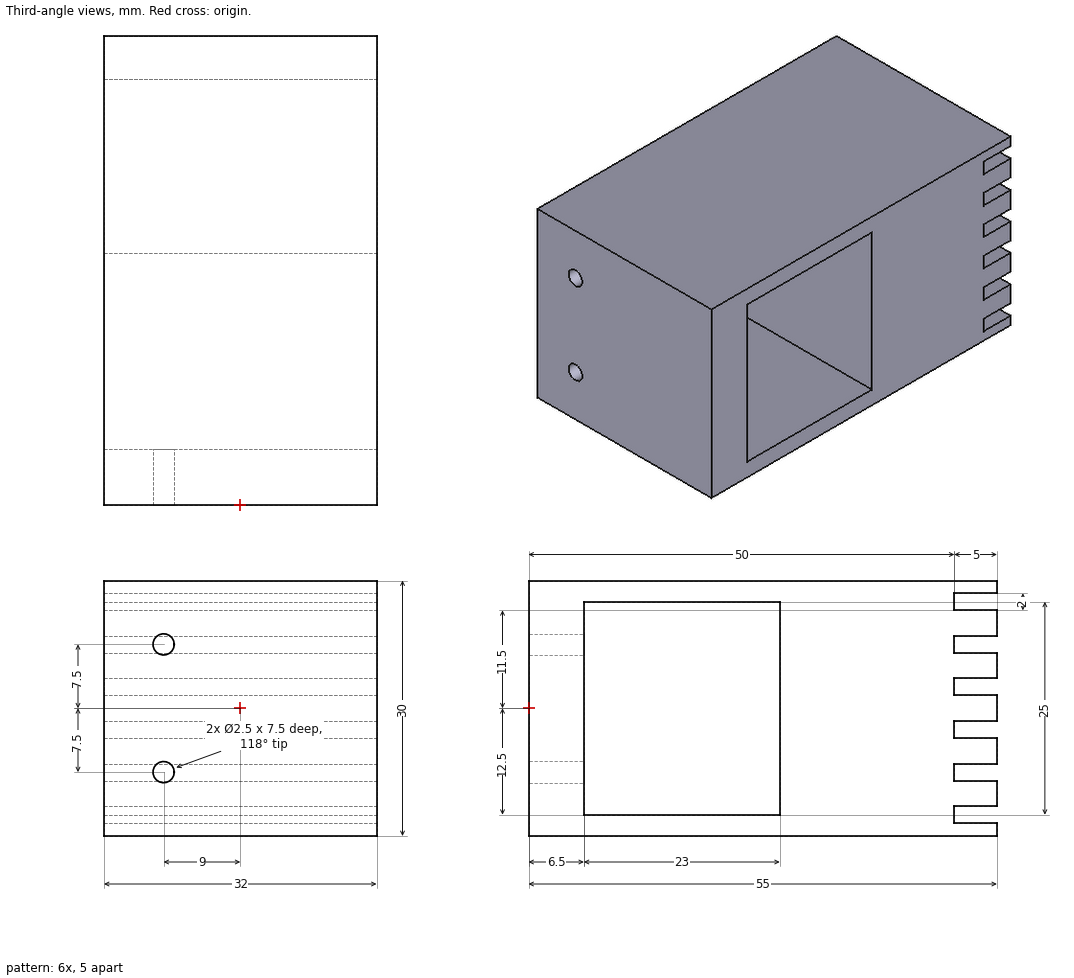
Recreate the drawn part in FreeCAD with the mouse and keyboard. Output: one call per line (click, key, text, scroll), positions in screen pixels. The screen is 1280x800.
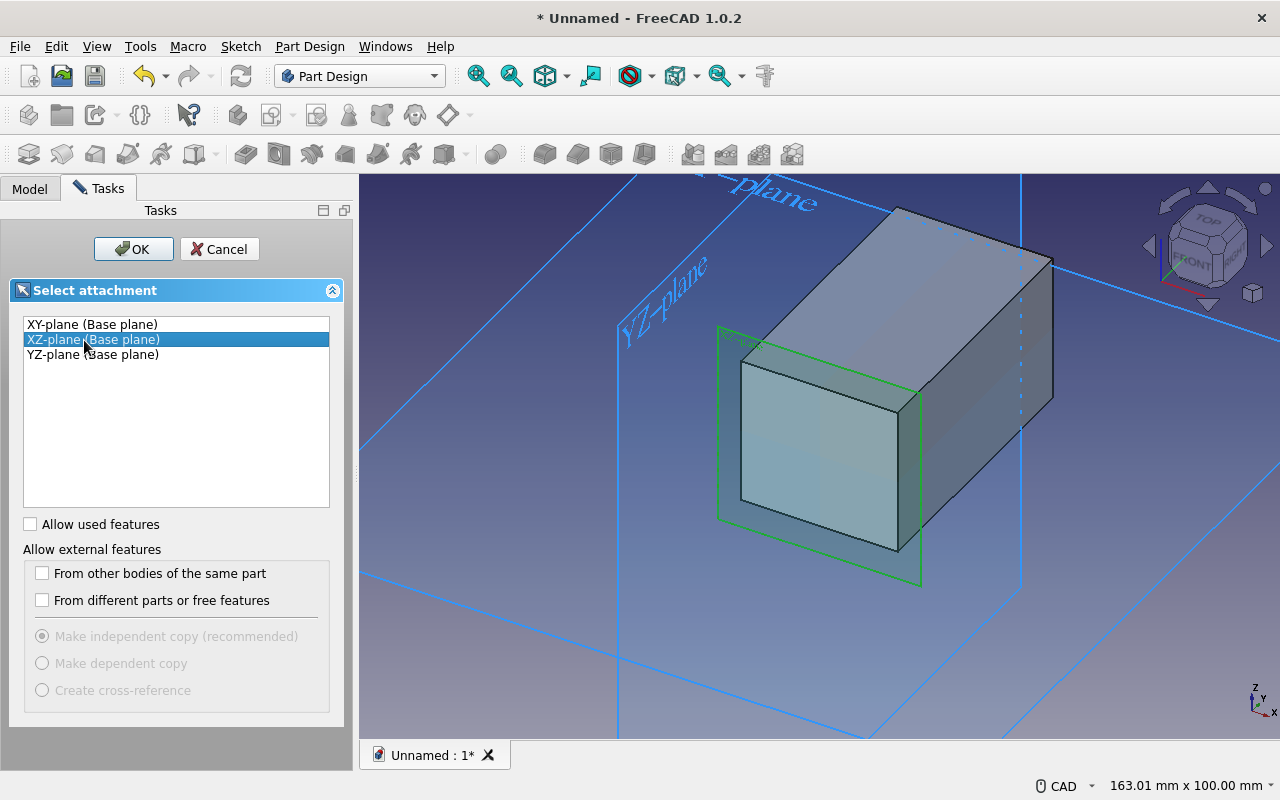
click(134, 249)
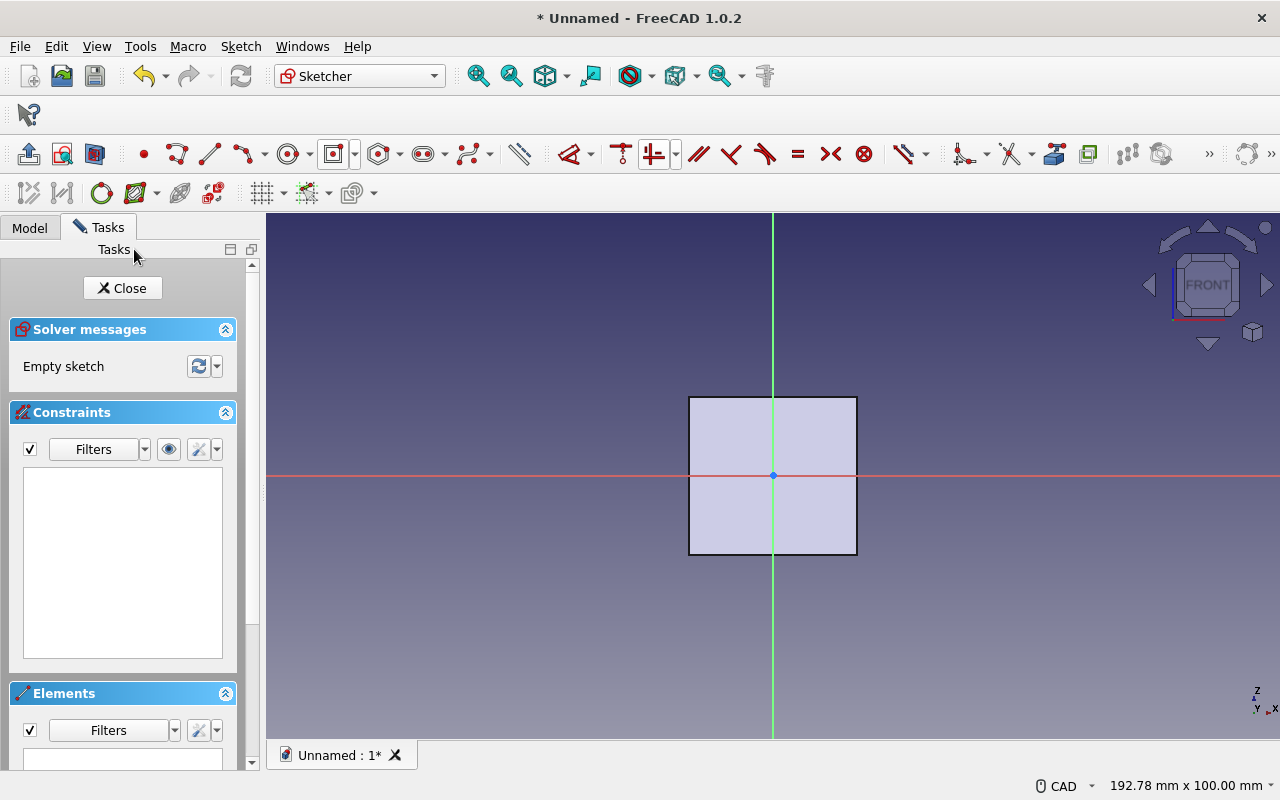
scroll(764, 476, up, 6)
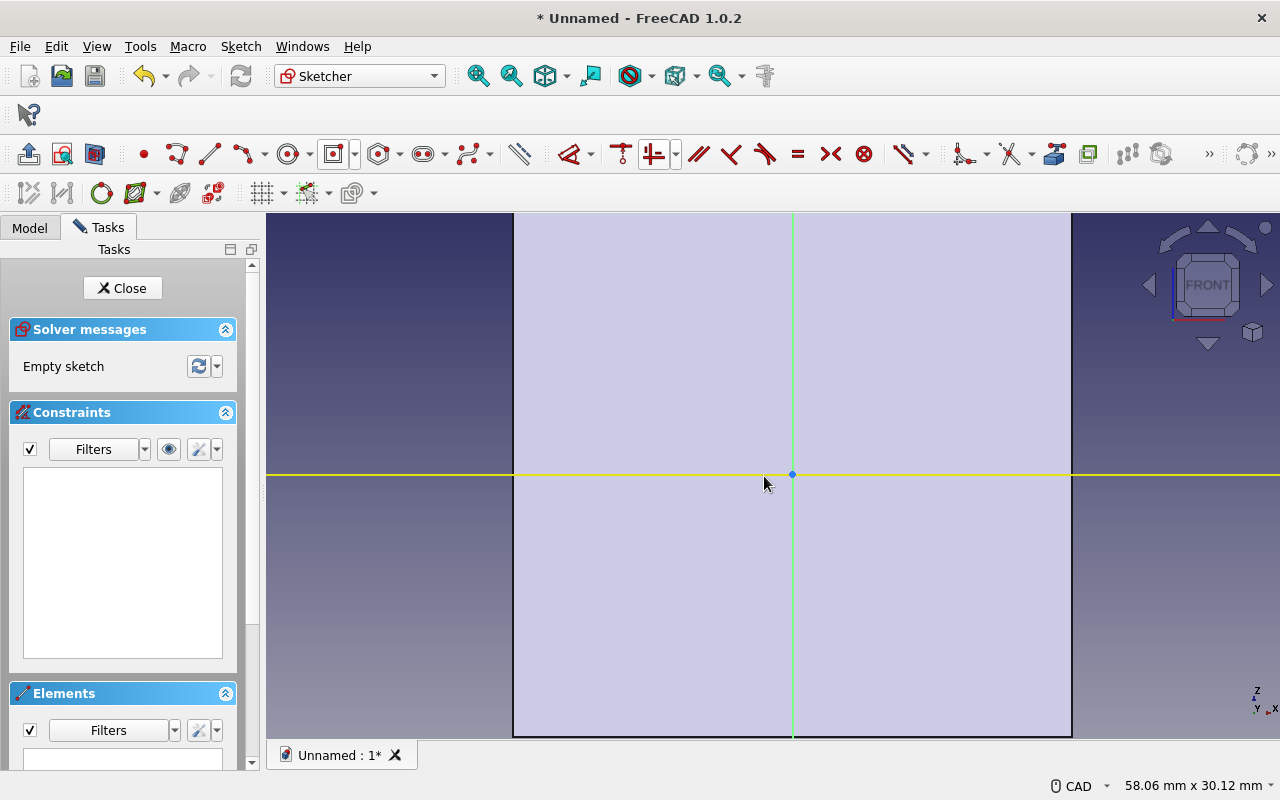
click(288, 154)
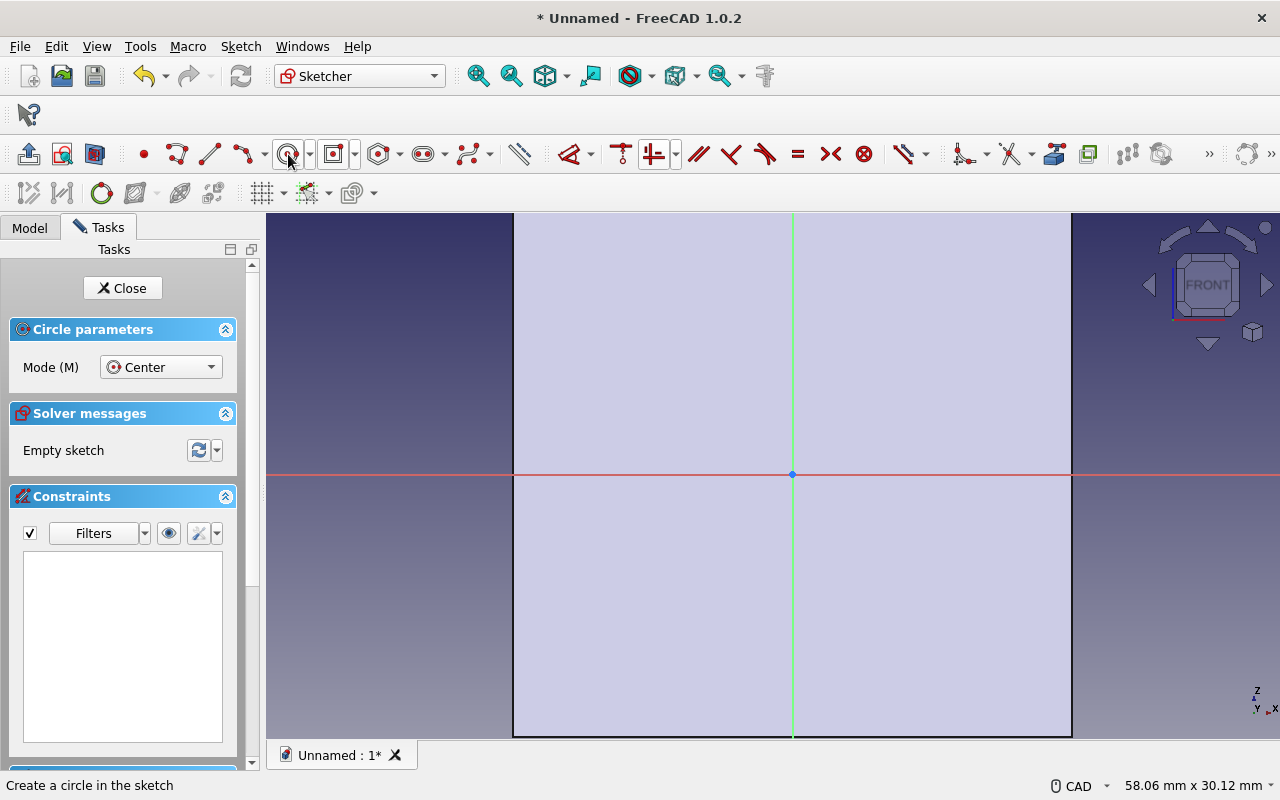
click(636, 606)
click(651, 590)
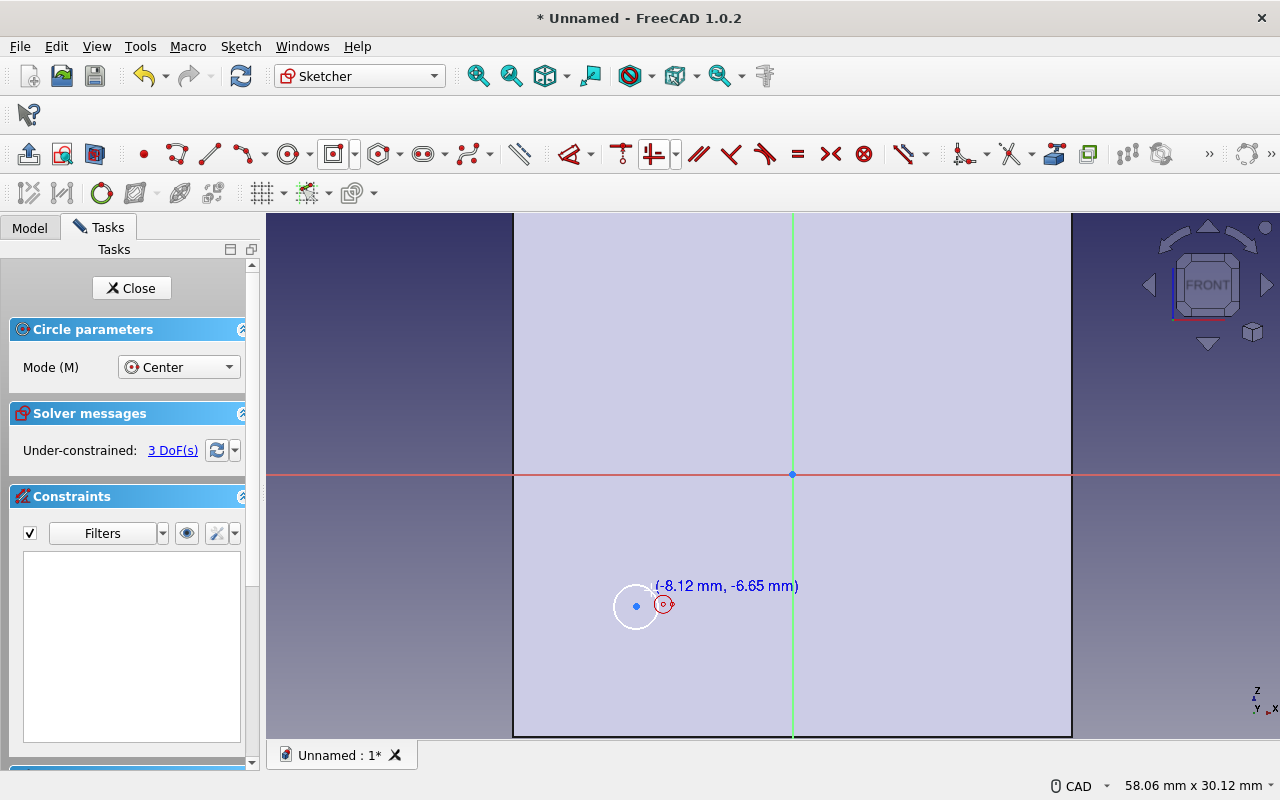
click(636, 344)
click(651, 328)
key(Escape)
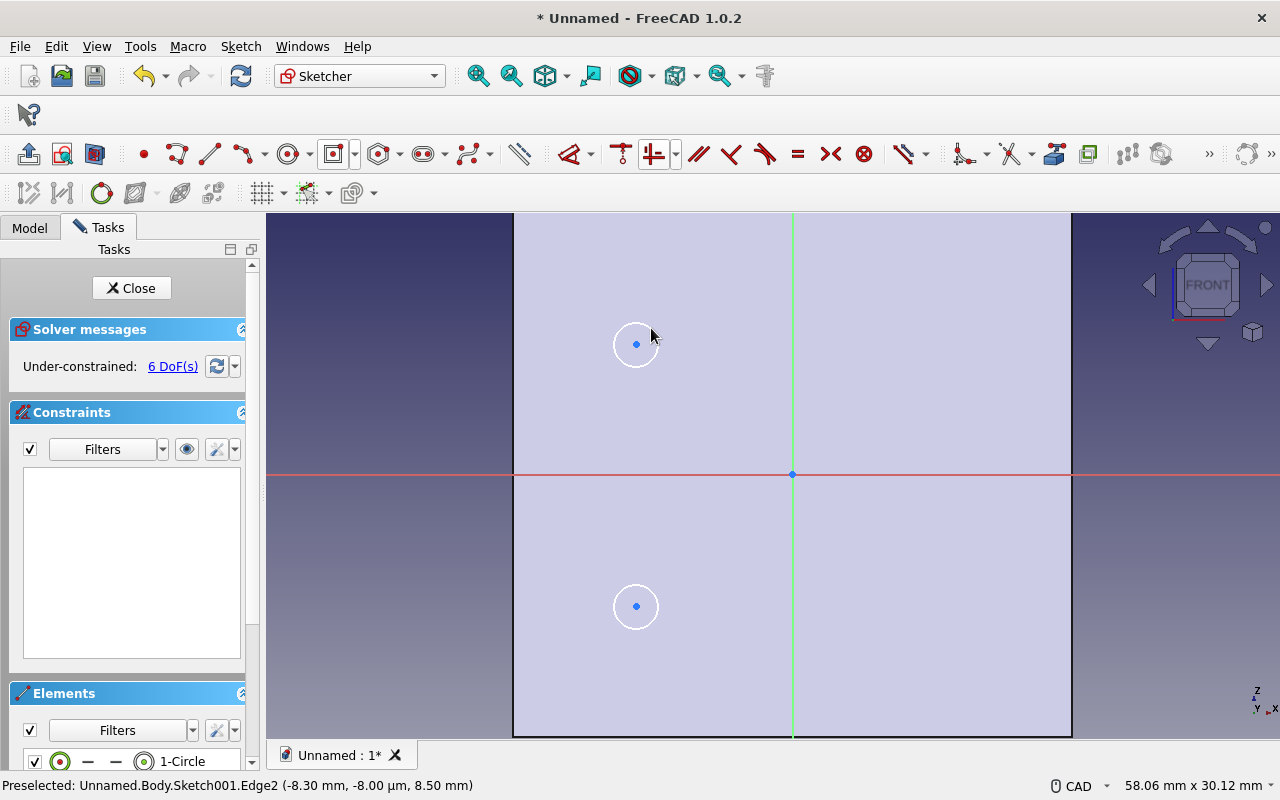
click(651, 591)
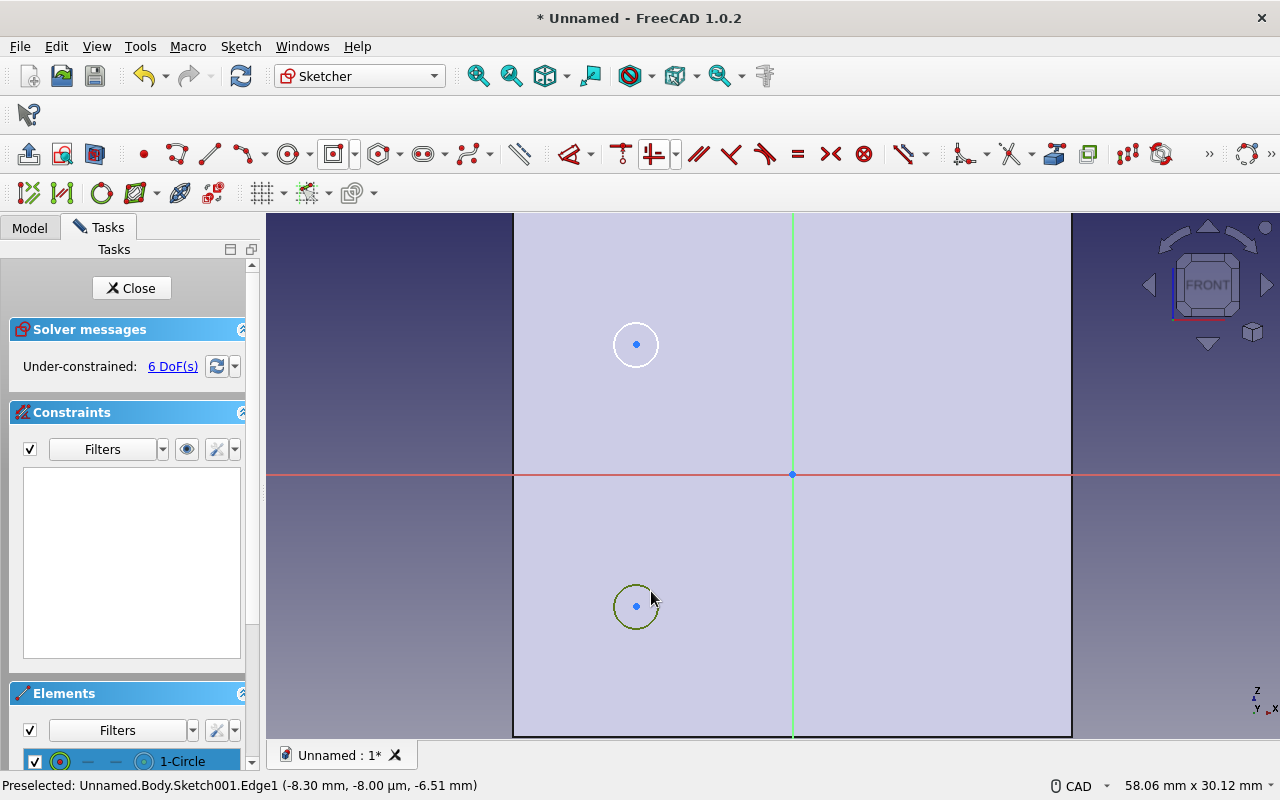
click(651, 329)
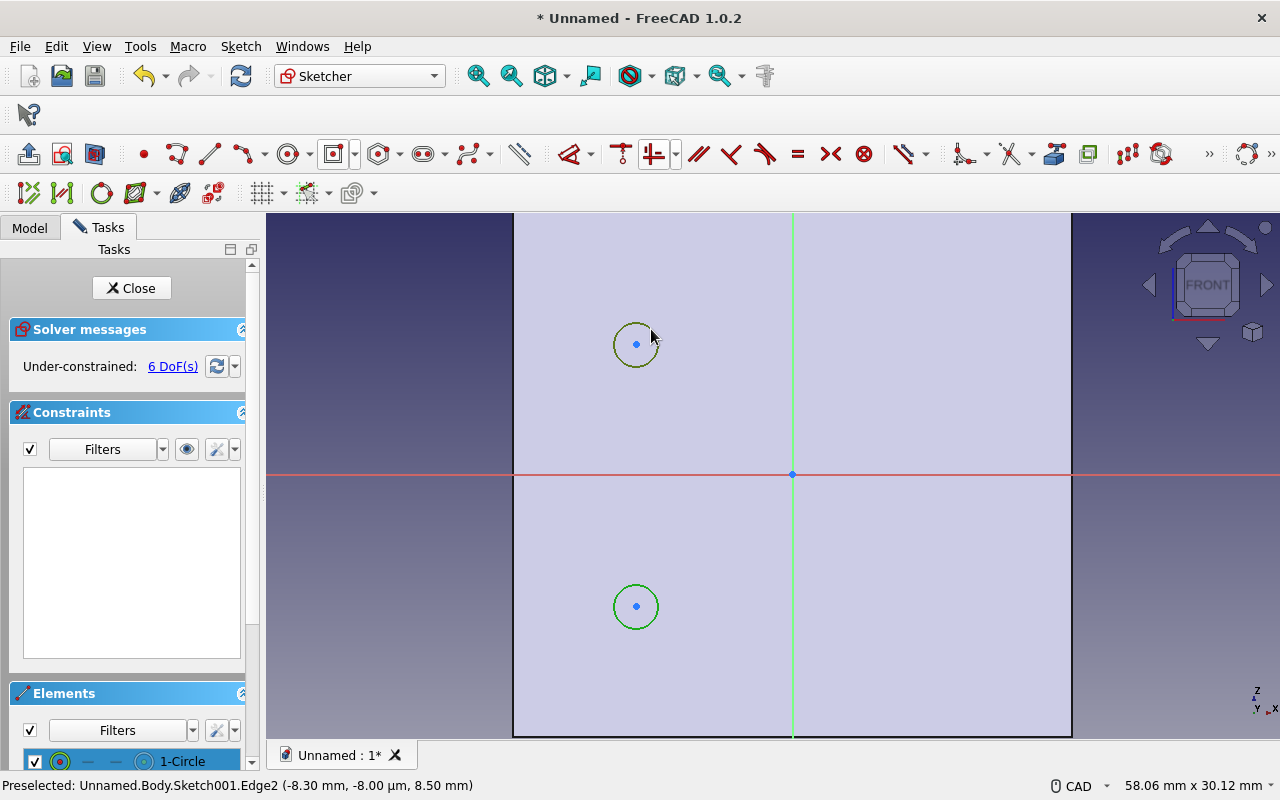
click(798, 154)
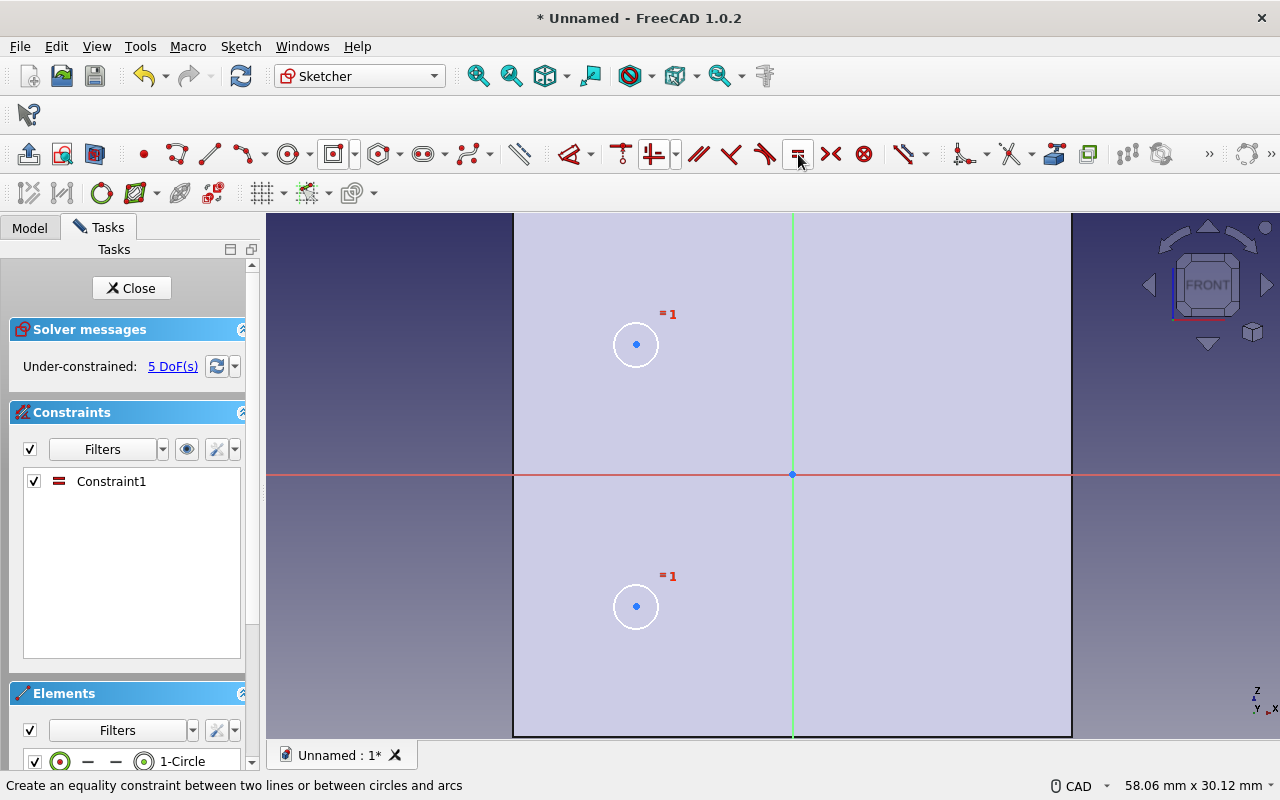
click(636, 607)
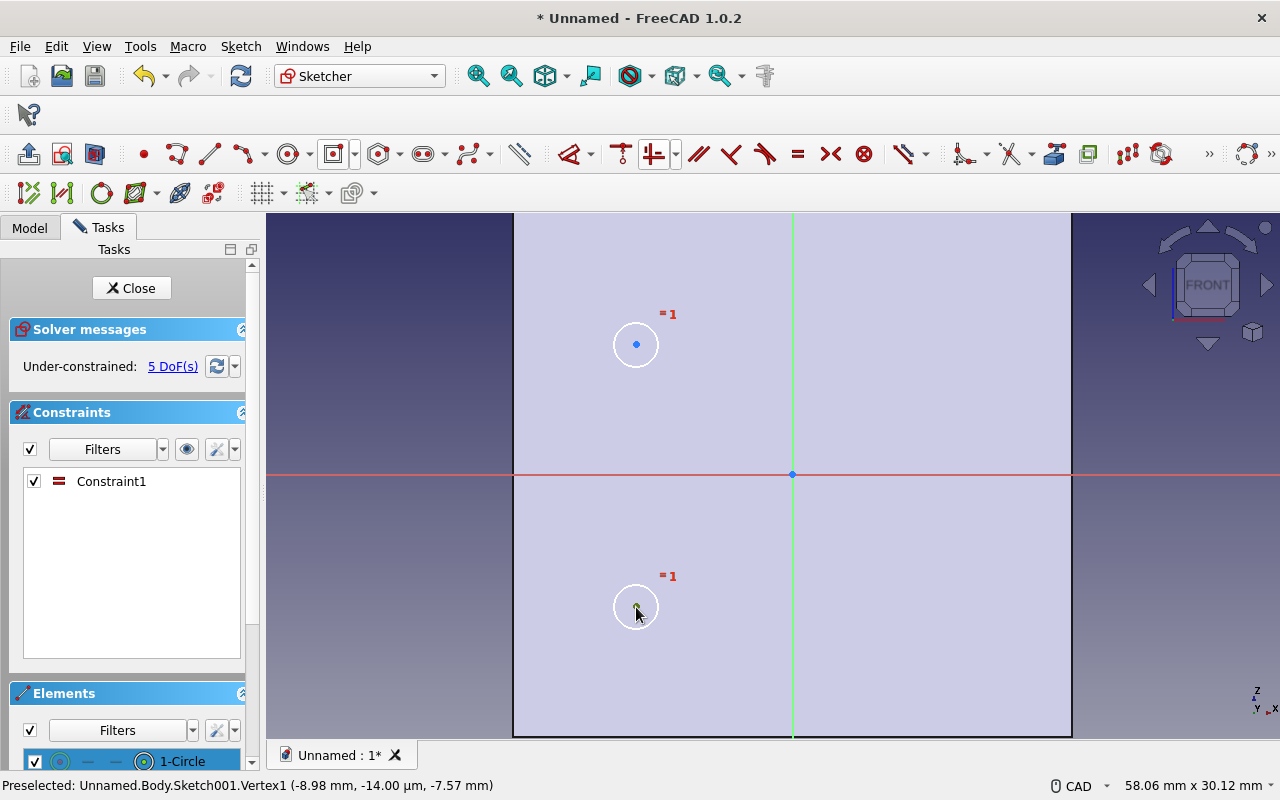
click(636, 345)